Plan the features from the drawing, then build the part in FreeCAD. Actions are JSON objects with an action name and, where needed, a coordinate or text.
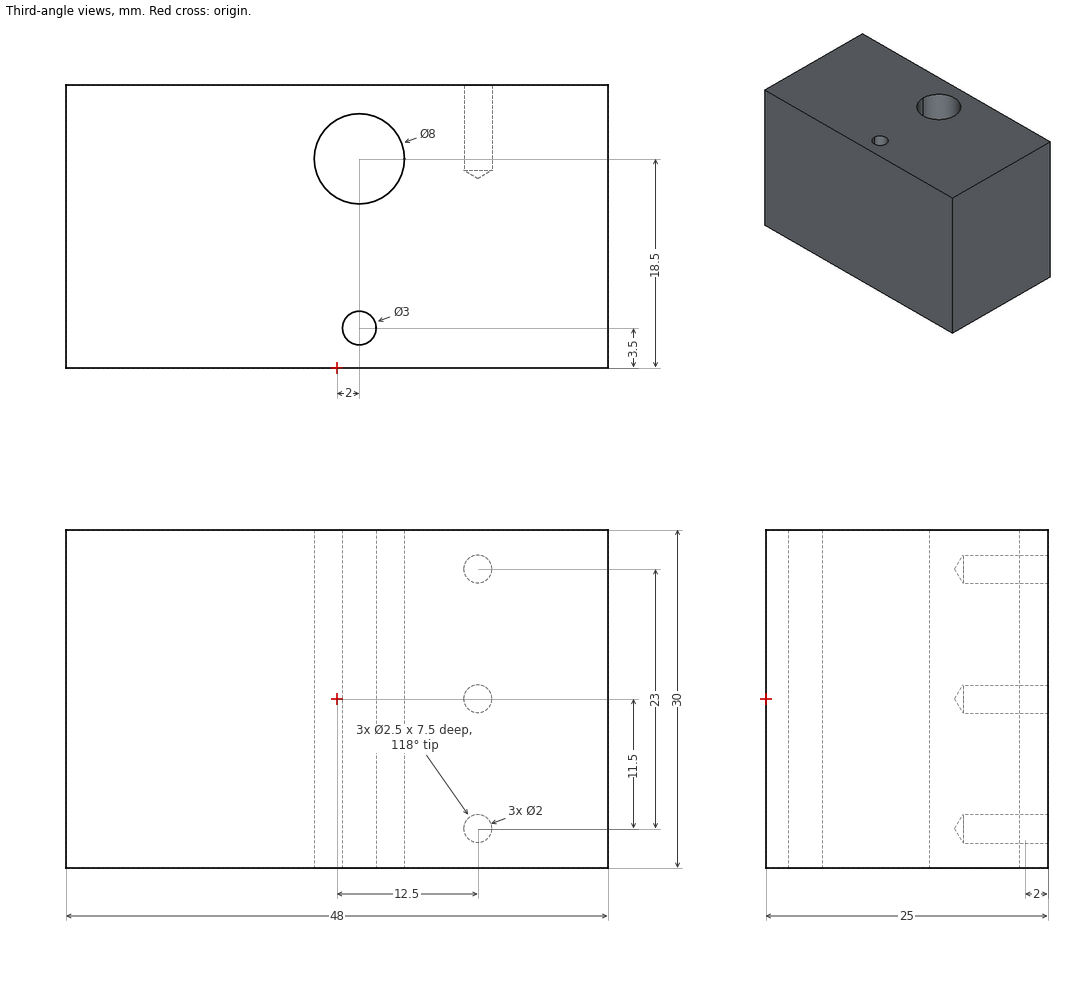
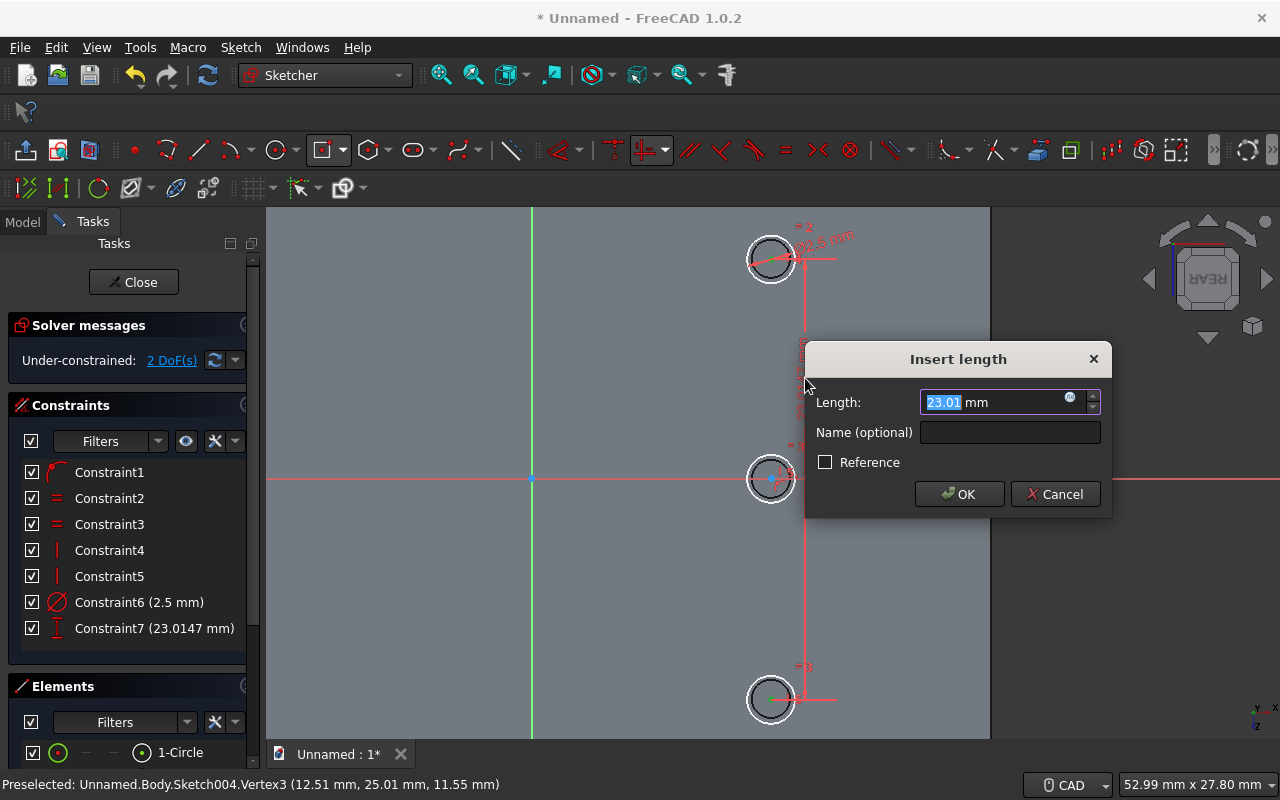
{"action": "type", "text": "23"}
{"action": "key", "text": "Return"}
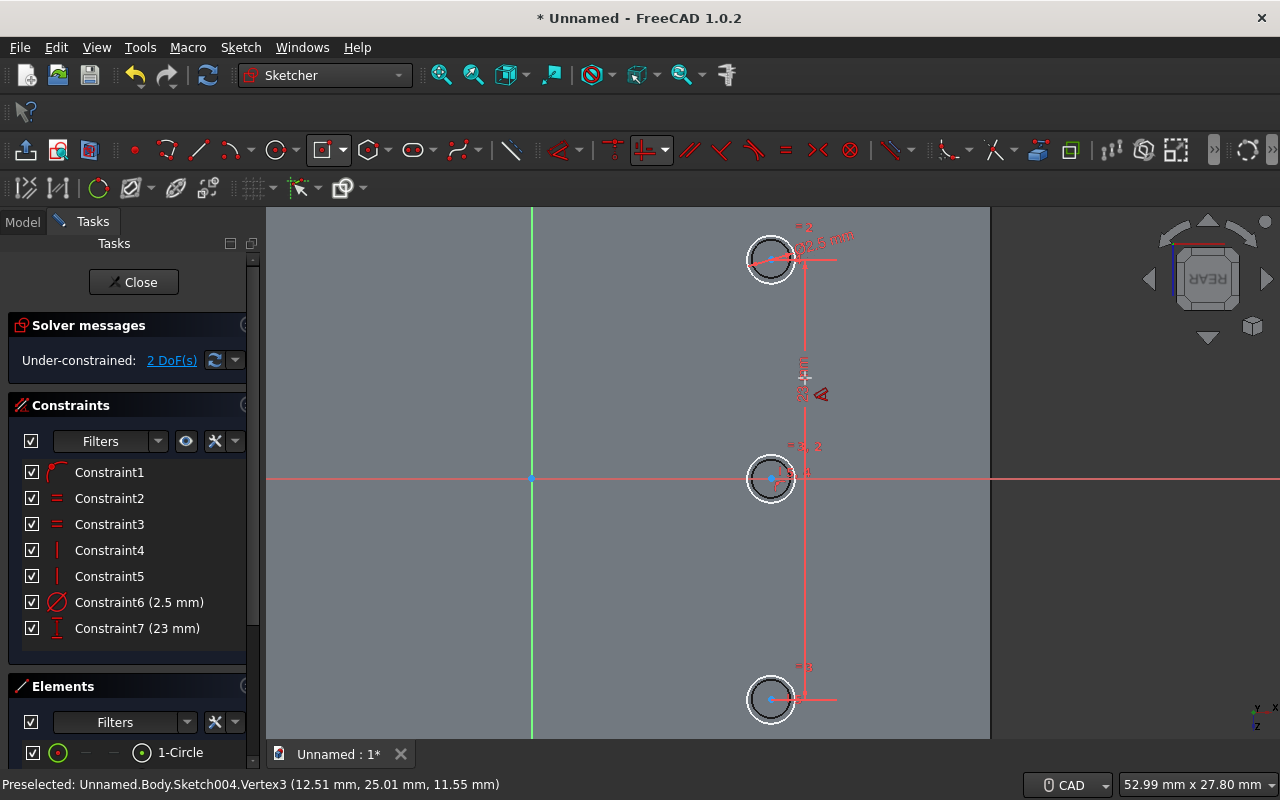
{"action": "left_click", "coordinate": [771, 260]}
{"action": "left_click", "coordinate": [651, 513]}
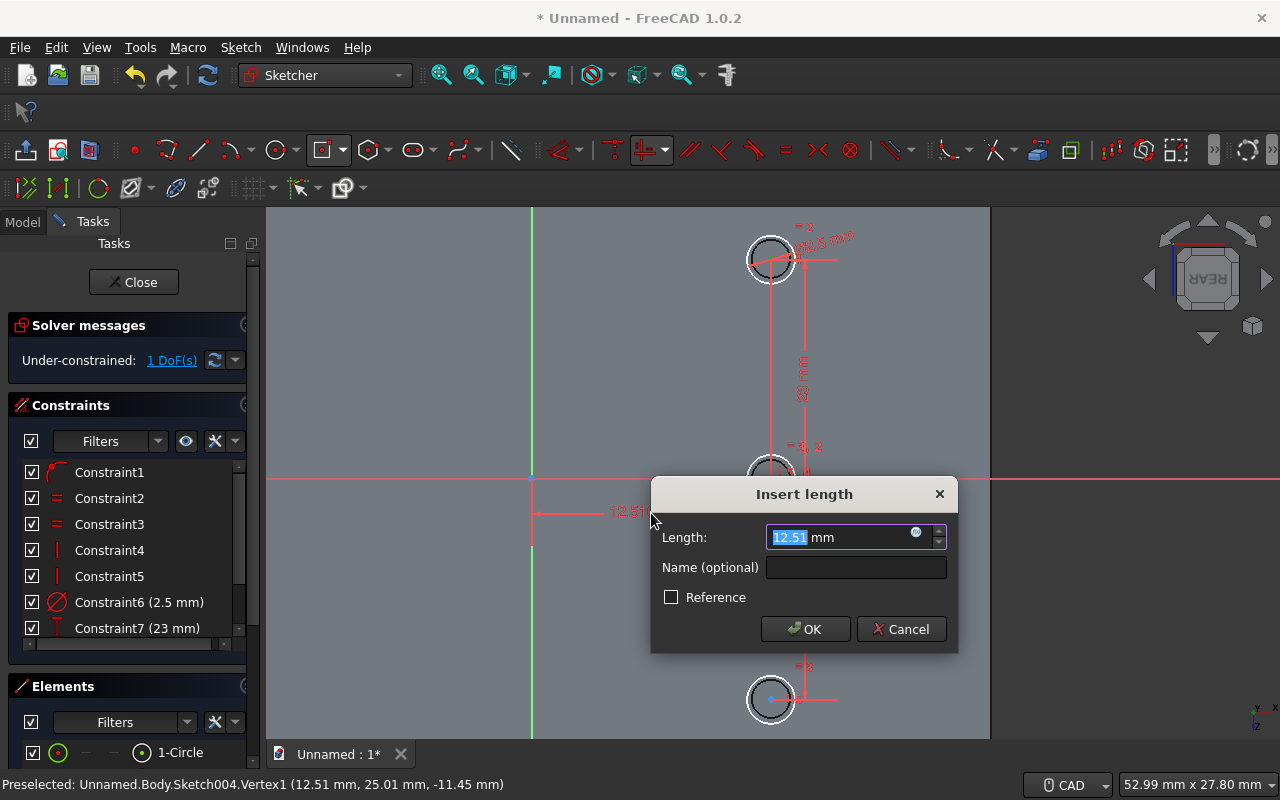
{"action": "type", "text": "12.5"}
{"action": "key", "text": "Return"}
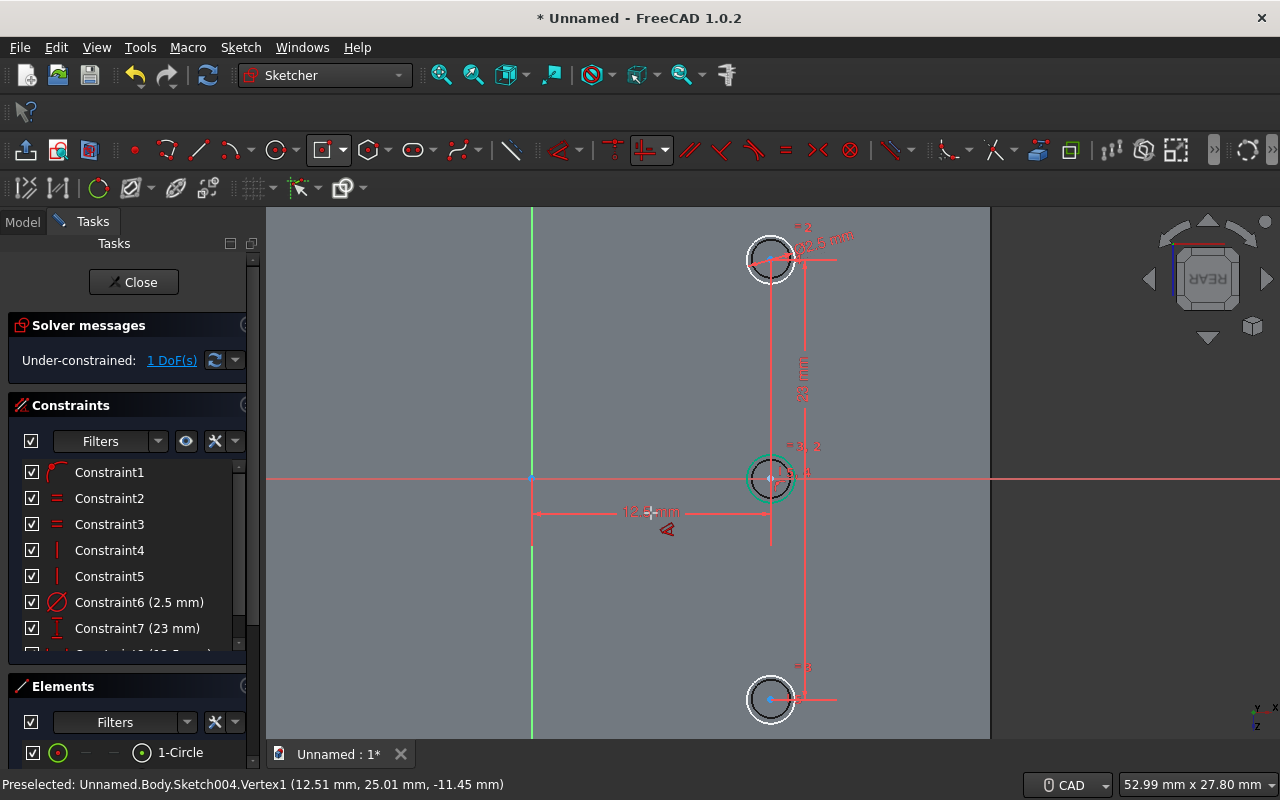
{"action": "left_click", "coordinate": [771, 260]}
{"action": "left_click", "coordinate": [498, 369]}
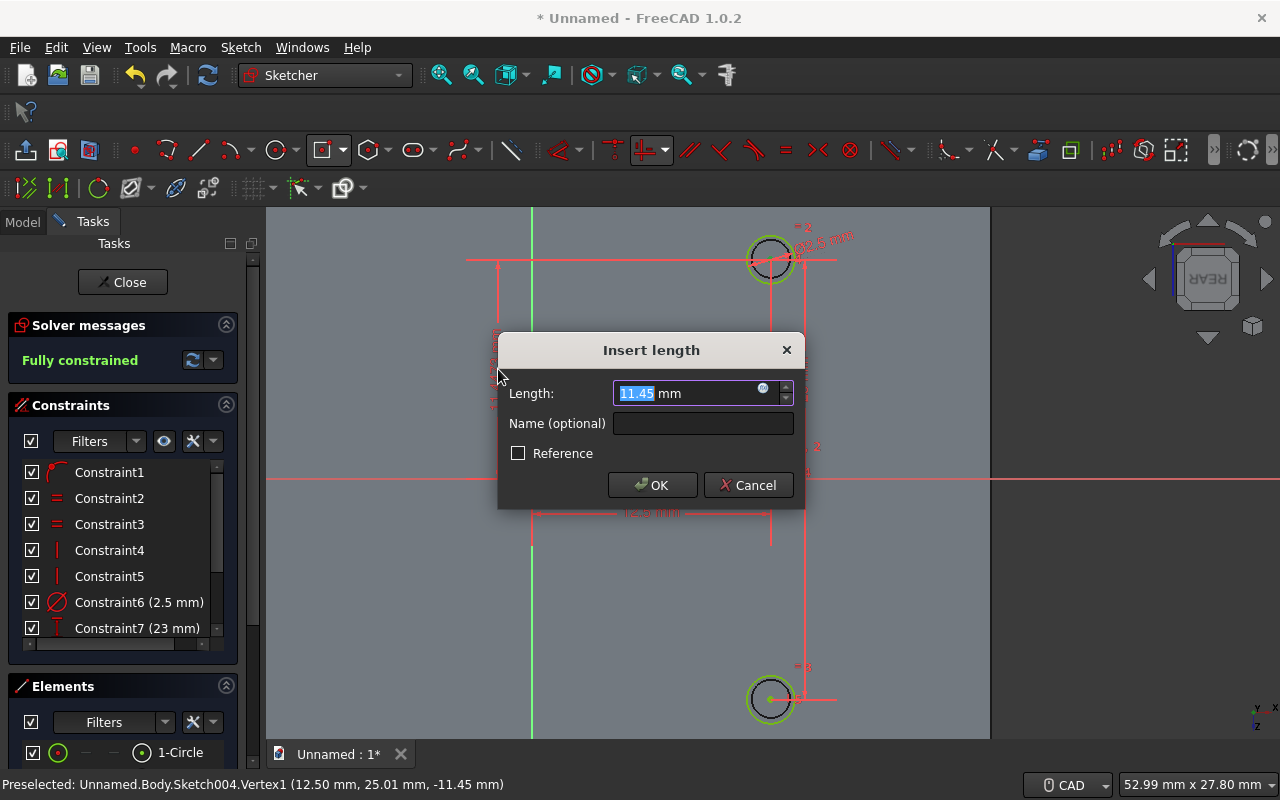
{"action": "type", "text": "11.5"}
{"action": "key", "text": "Return"}
{"action": "key", "text": "Escape"}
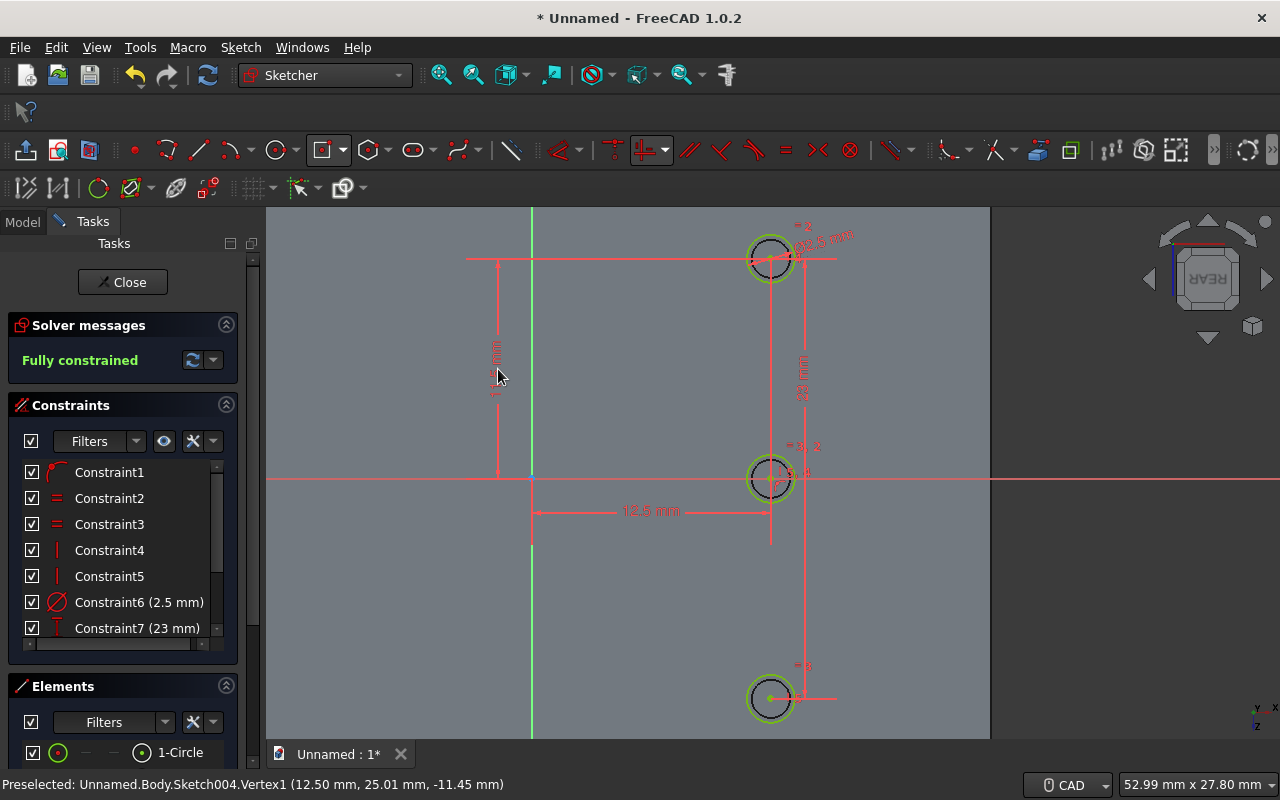
{"action": "left_click", "coordinate": [123, 282]}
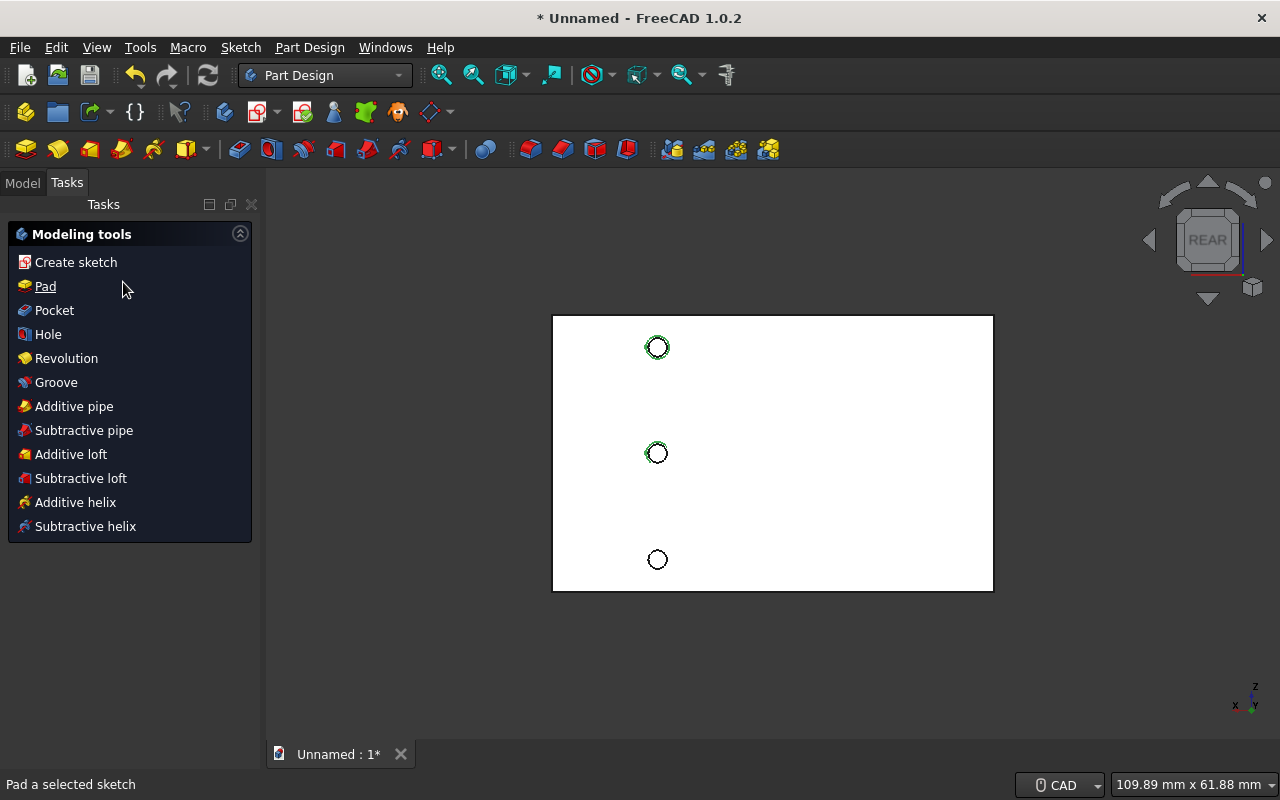
{"action": "left_click", "coordinate": [272, 150]}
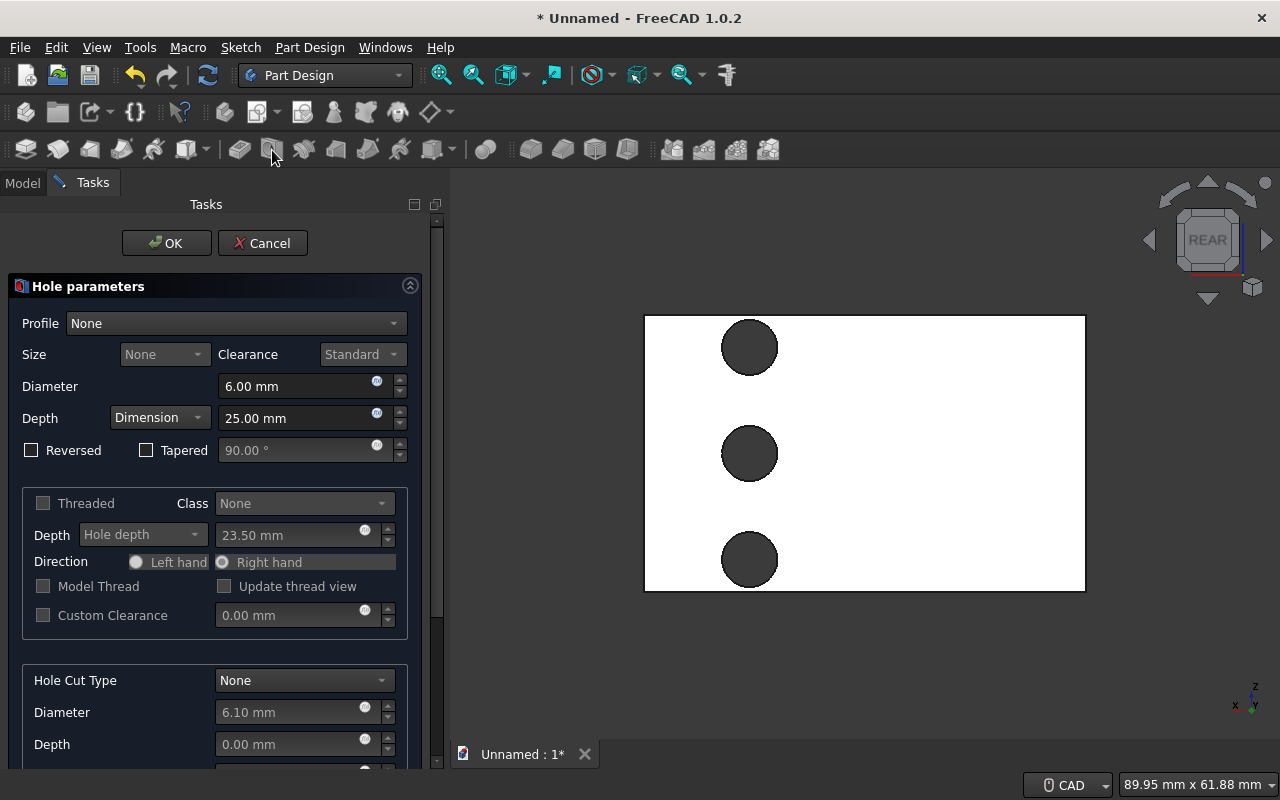
{"action": "triple_click", "coordinate": [305, 386]}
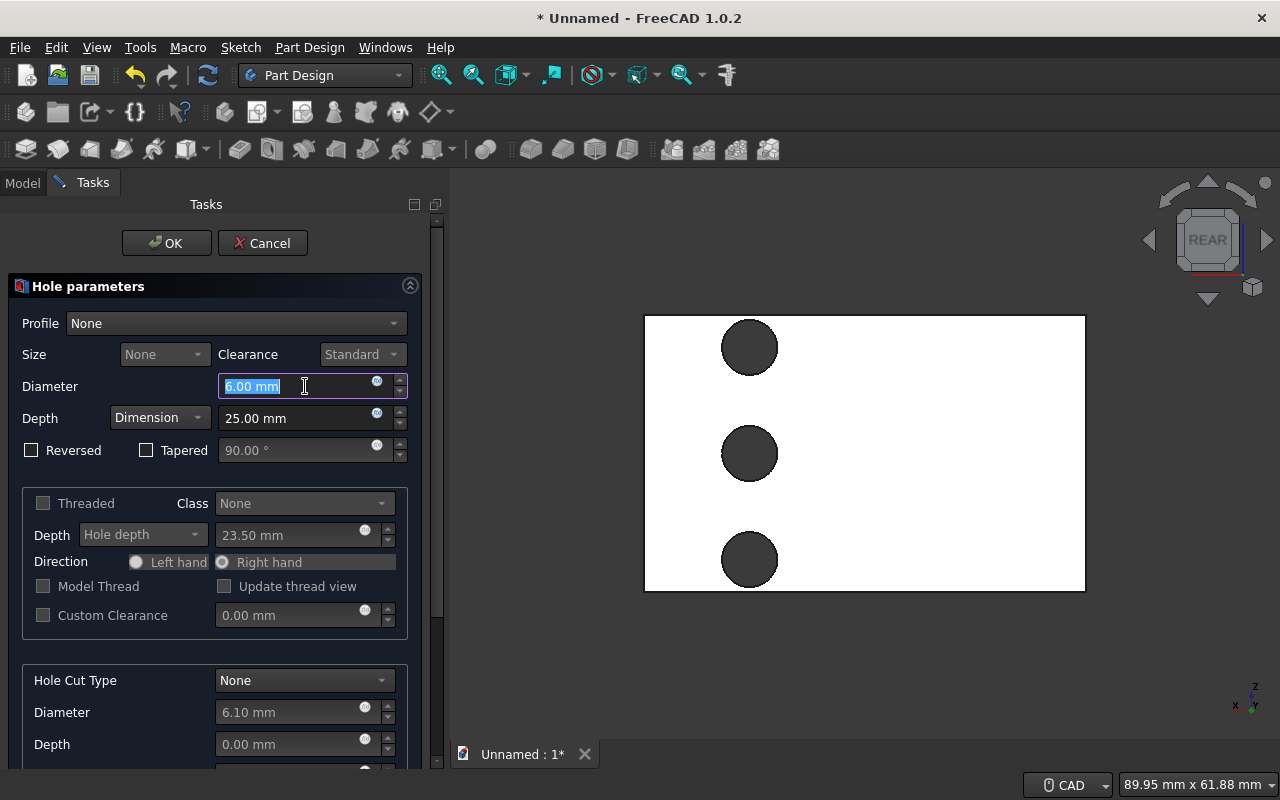
{"action": "type", "text": "2.5"}
{"action": "key", "text": "Tab"}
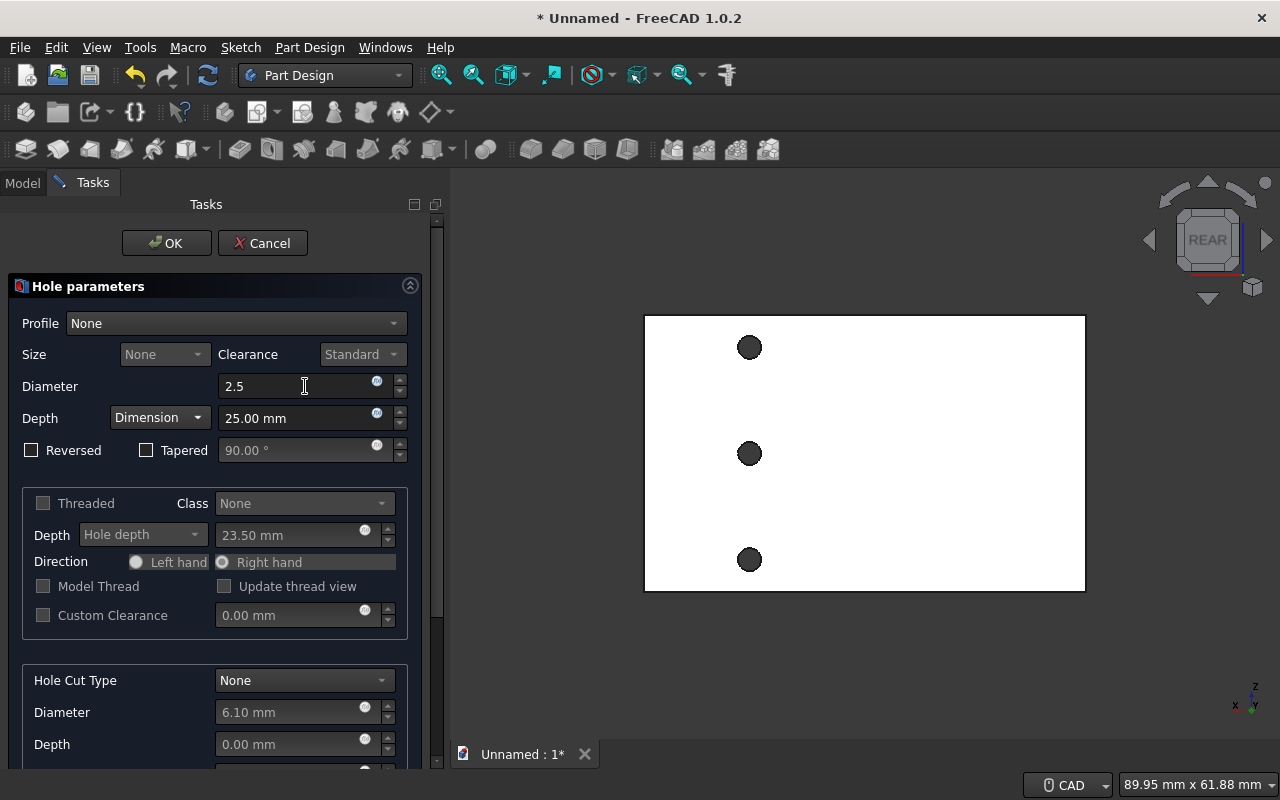
{"action": "triple_click", "coordinate": [305, 418]}